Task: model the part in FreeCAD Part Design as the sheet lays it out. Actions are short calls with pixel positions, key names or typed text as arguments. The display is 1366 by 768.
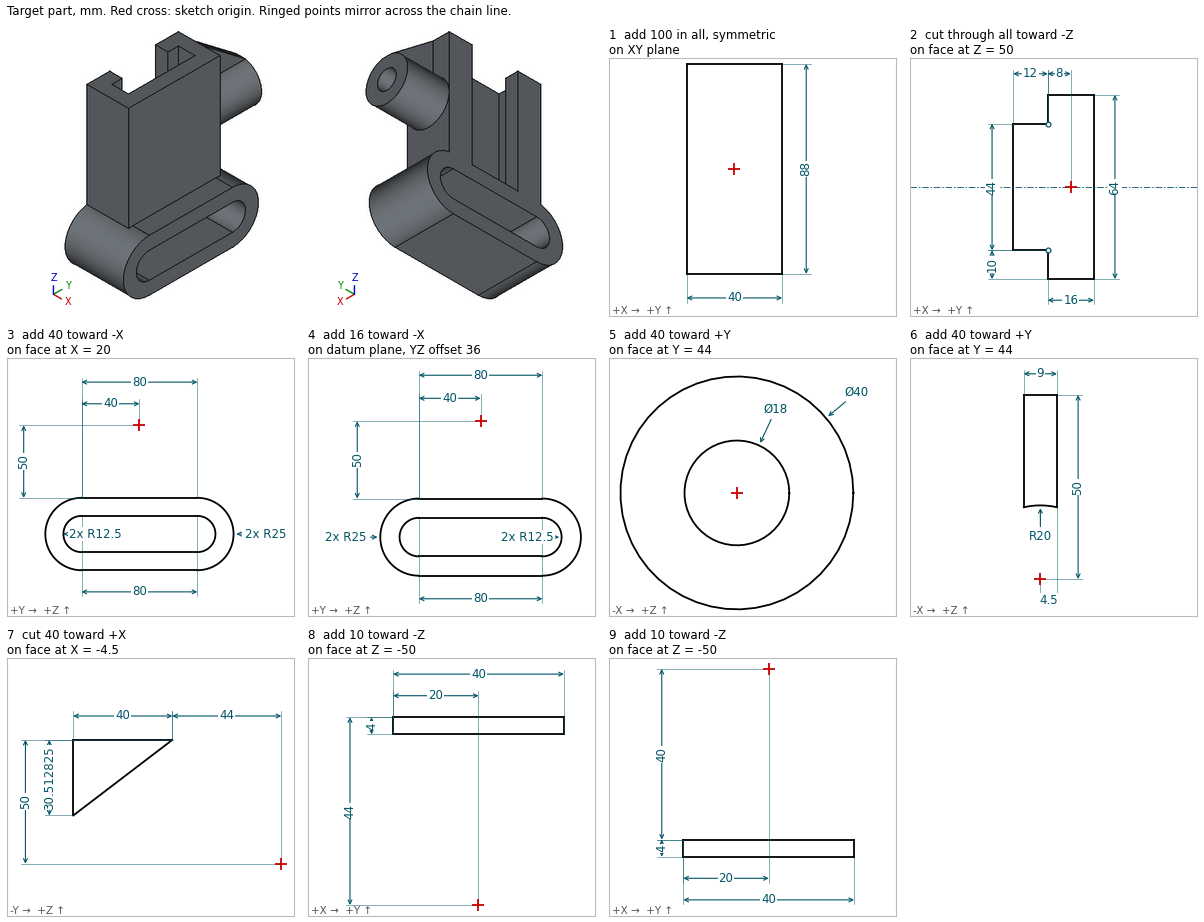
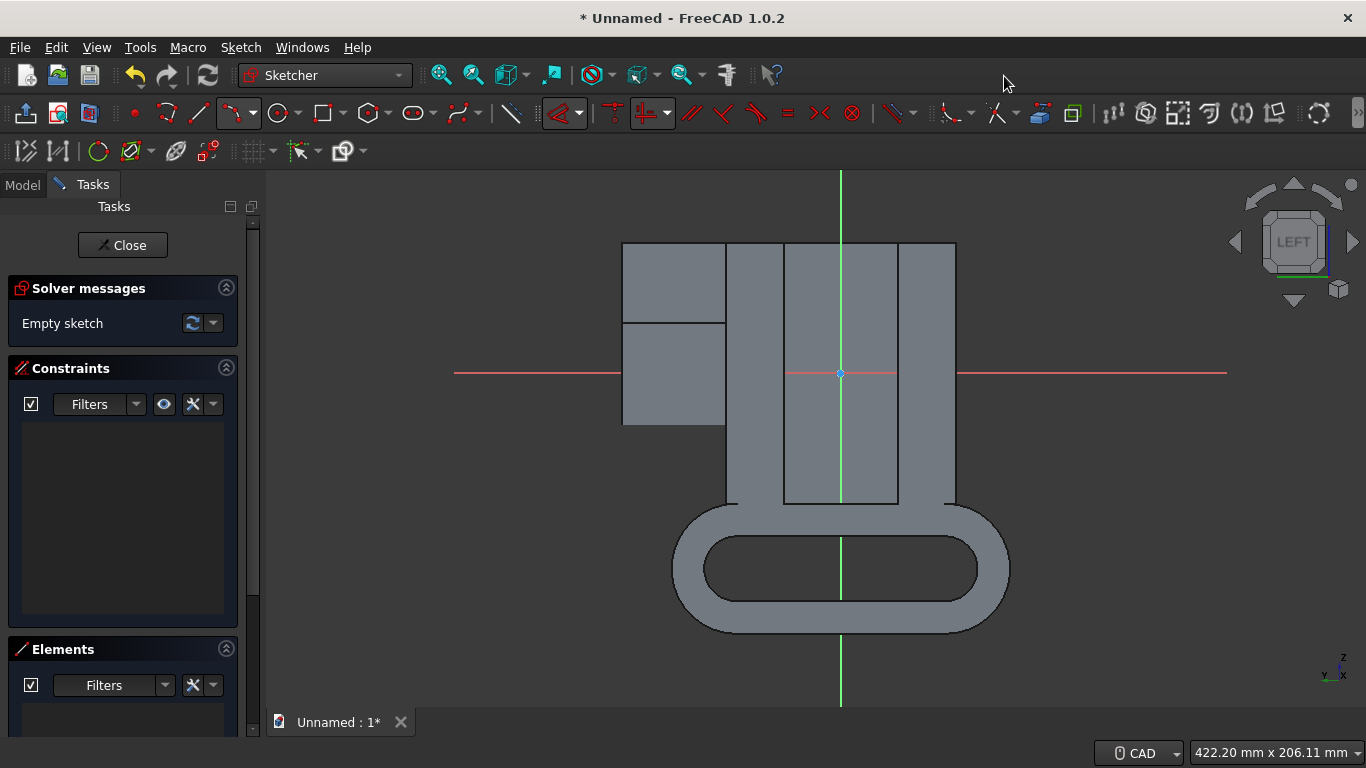
scroll(722, 232, up, 5)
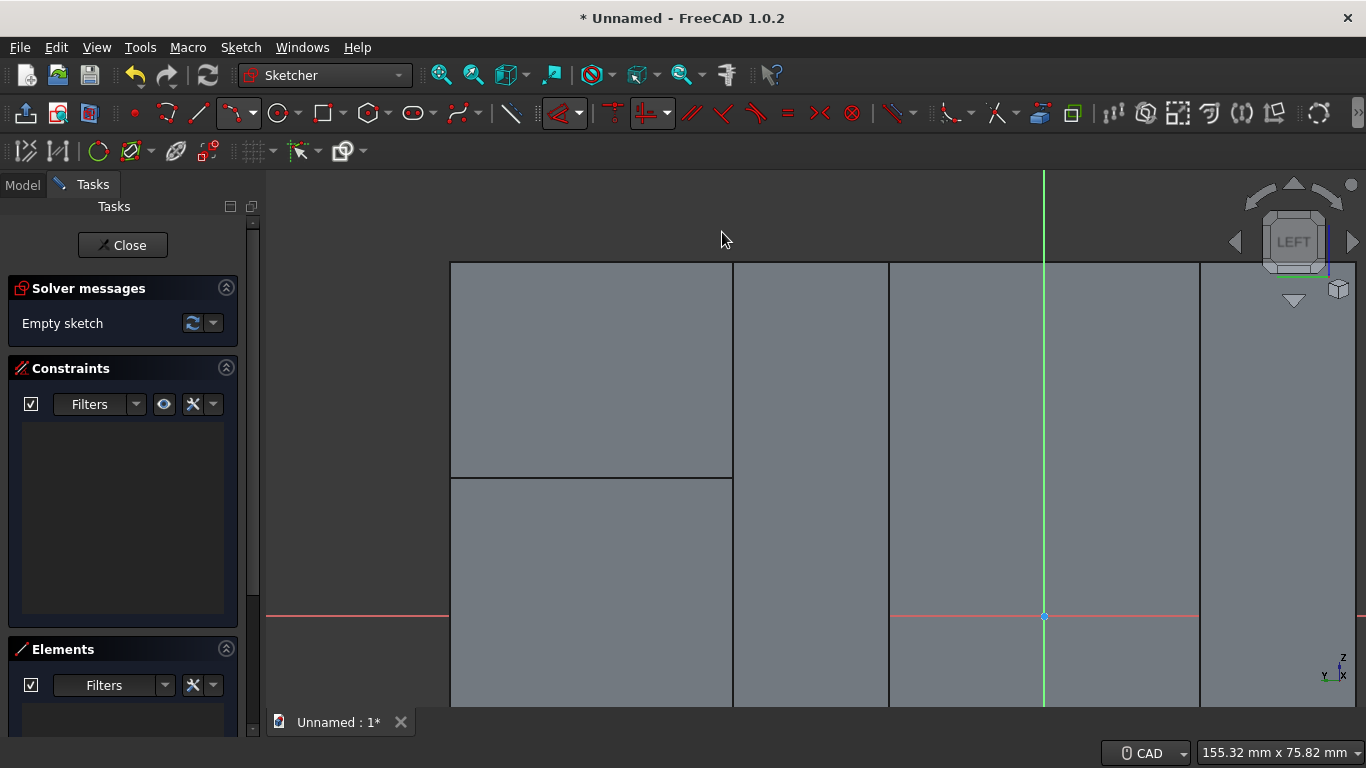
key(g)
key(m)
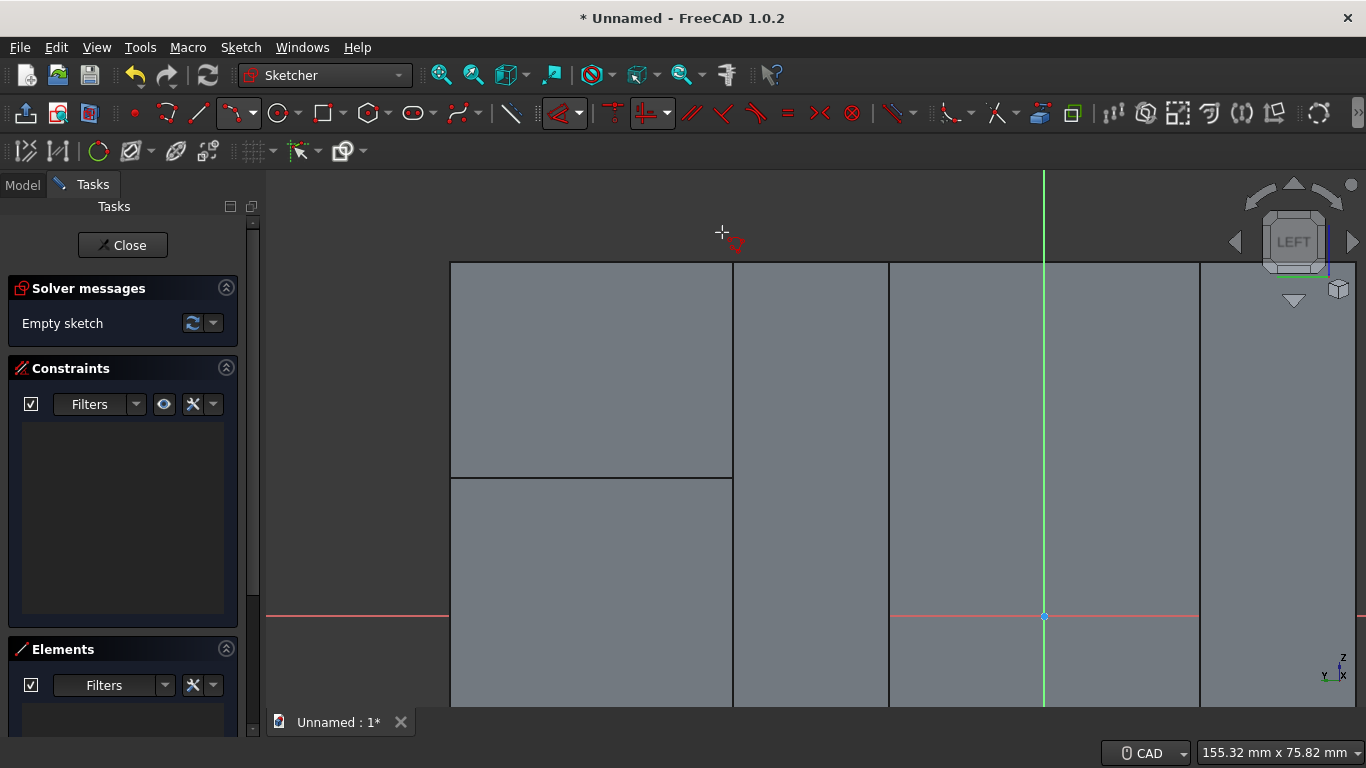
click(733, 262)
click(450, 262)
click(450, 478)
click(733, 263)
key(Escape)
key(Escape)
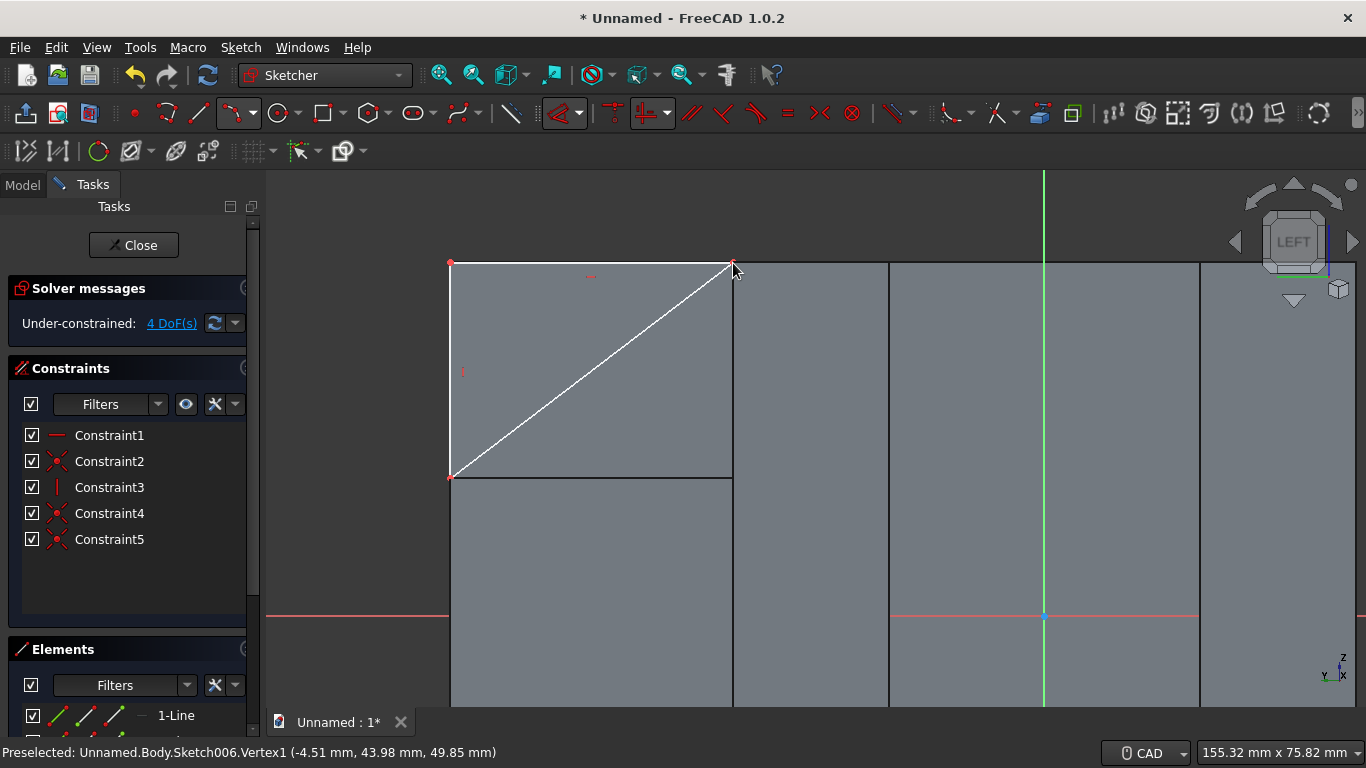
click(648, 263)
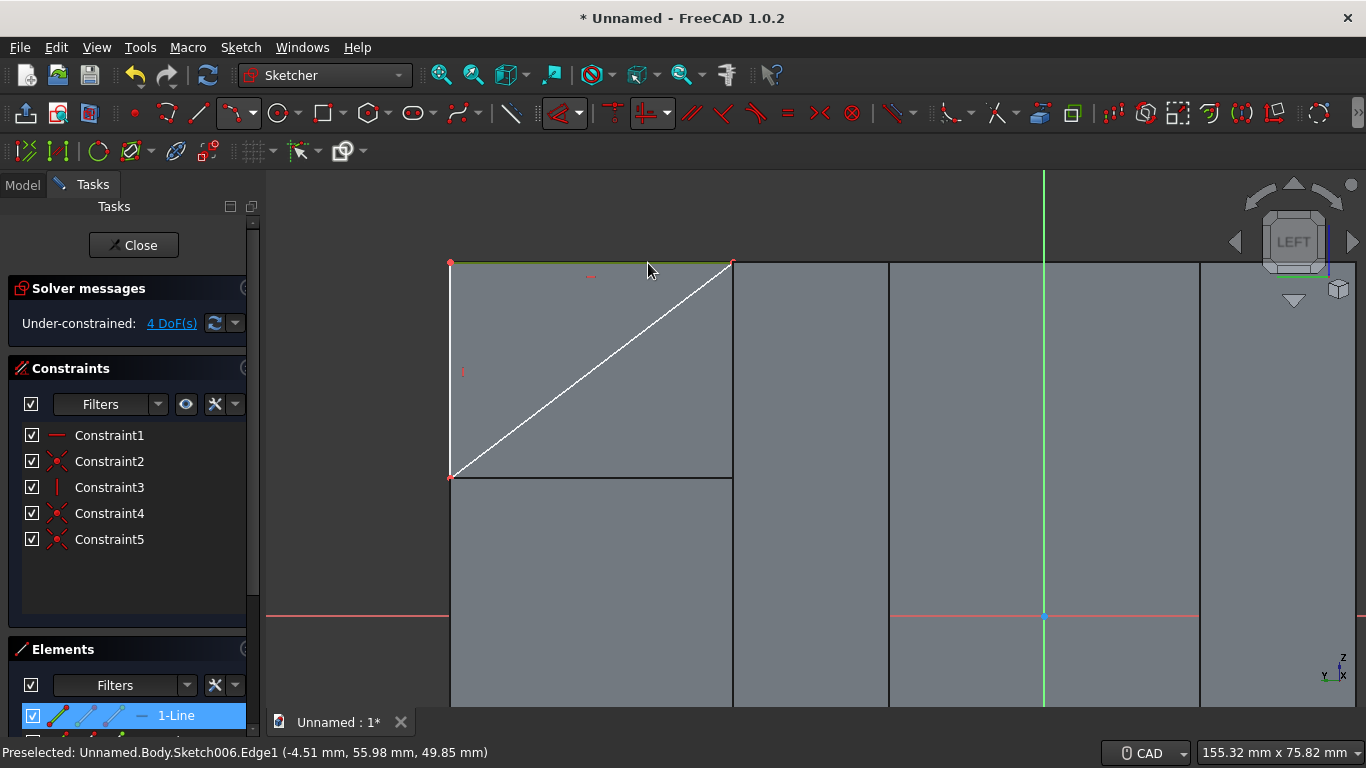
key(l)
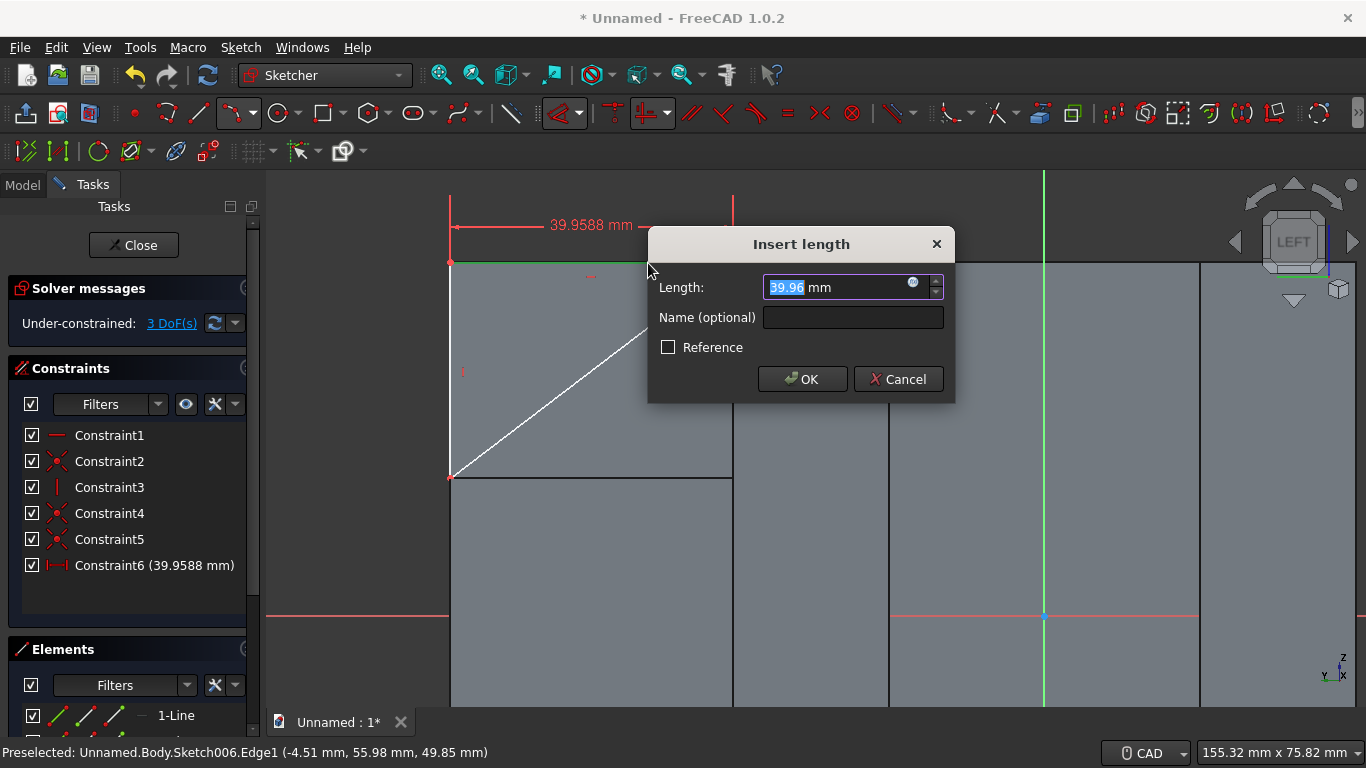
text(40)
key(Return)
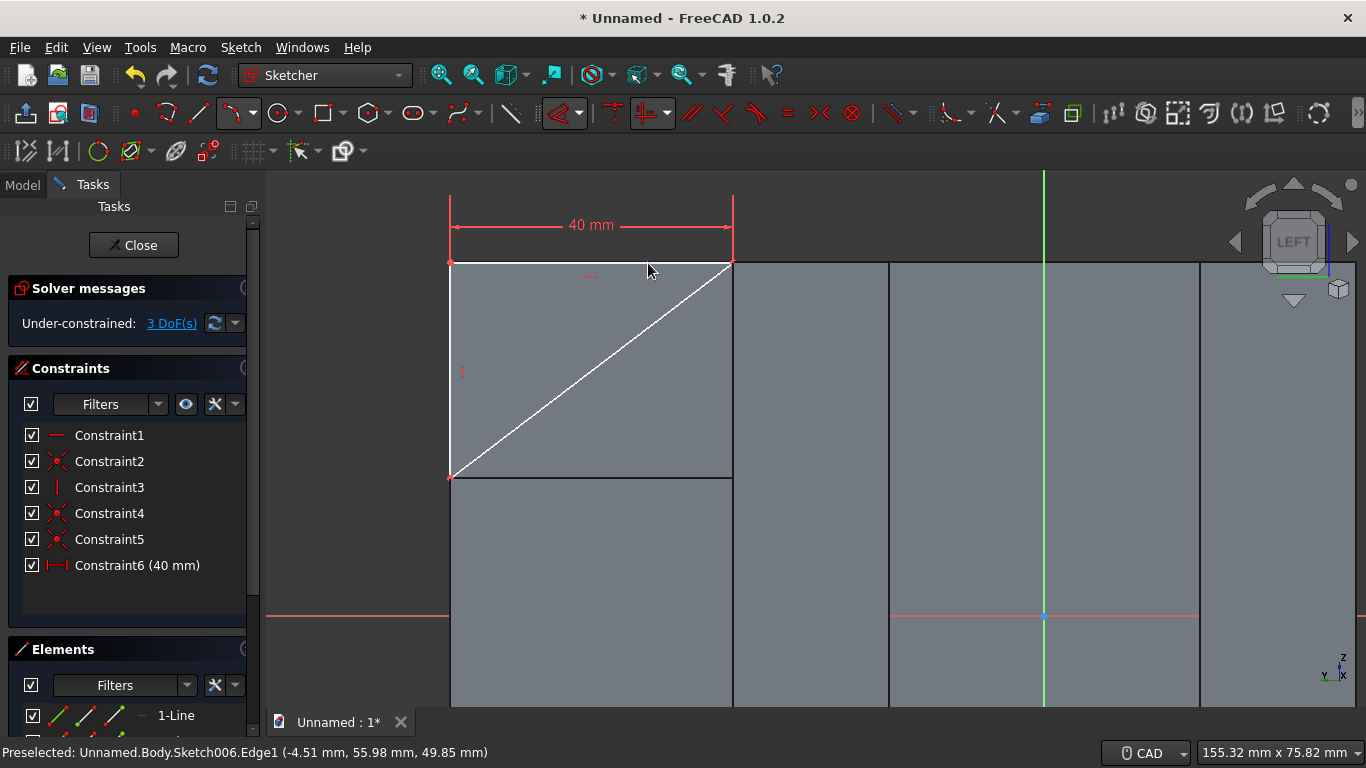
click(733, 263)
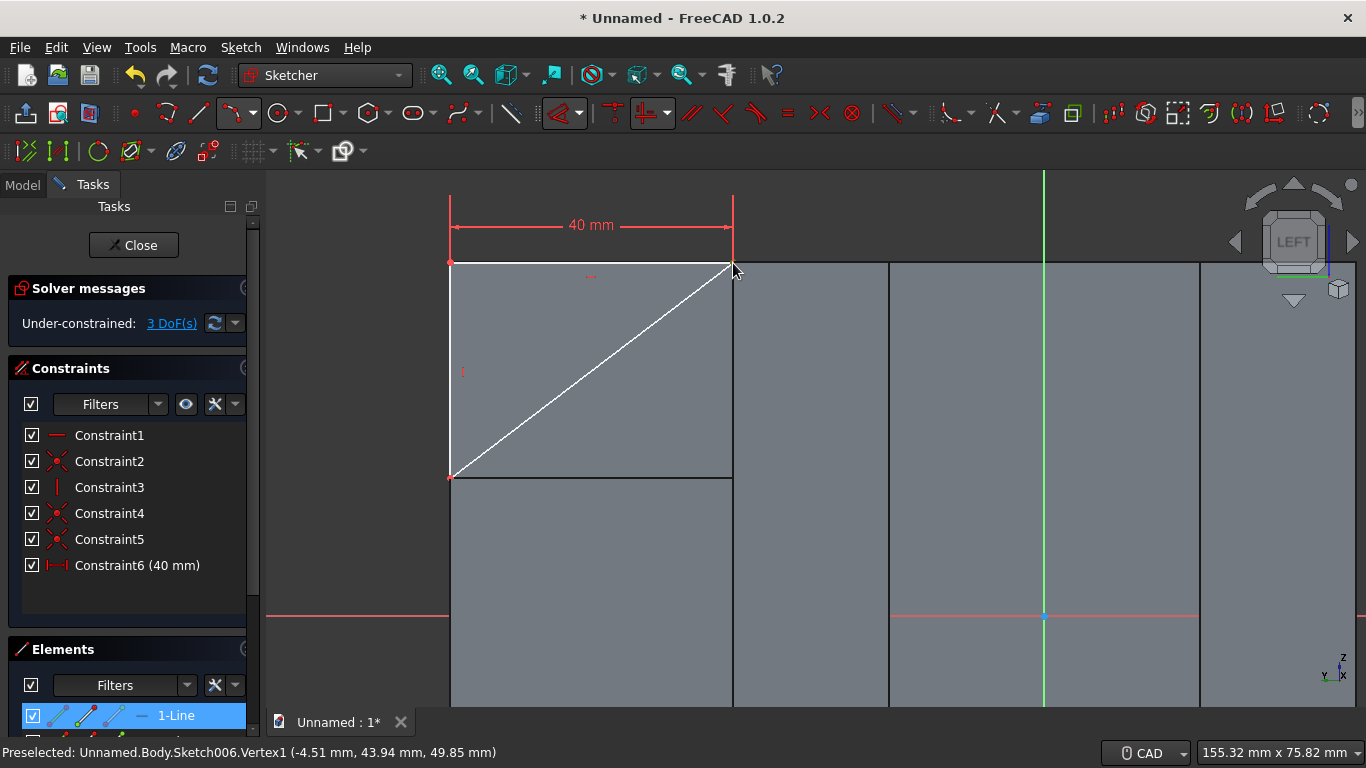
key(l)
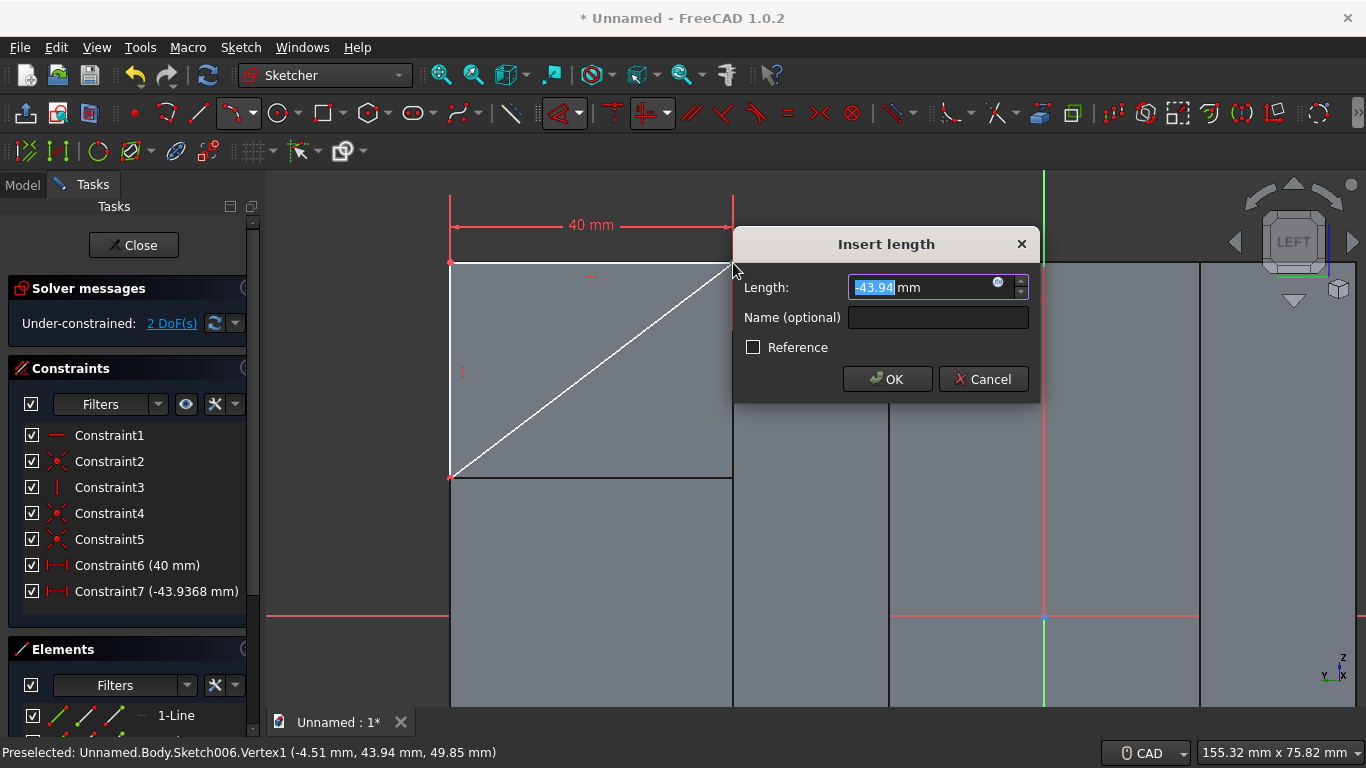
text(-44)
key(Return)